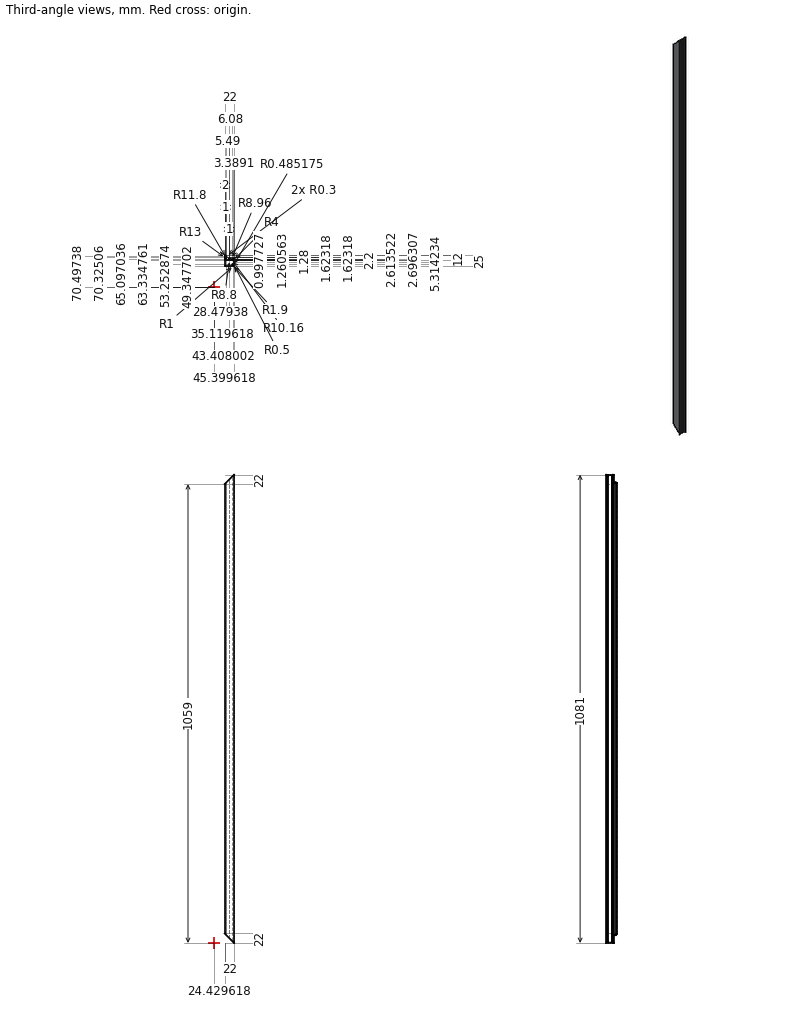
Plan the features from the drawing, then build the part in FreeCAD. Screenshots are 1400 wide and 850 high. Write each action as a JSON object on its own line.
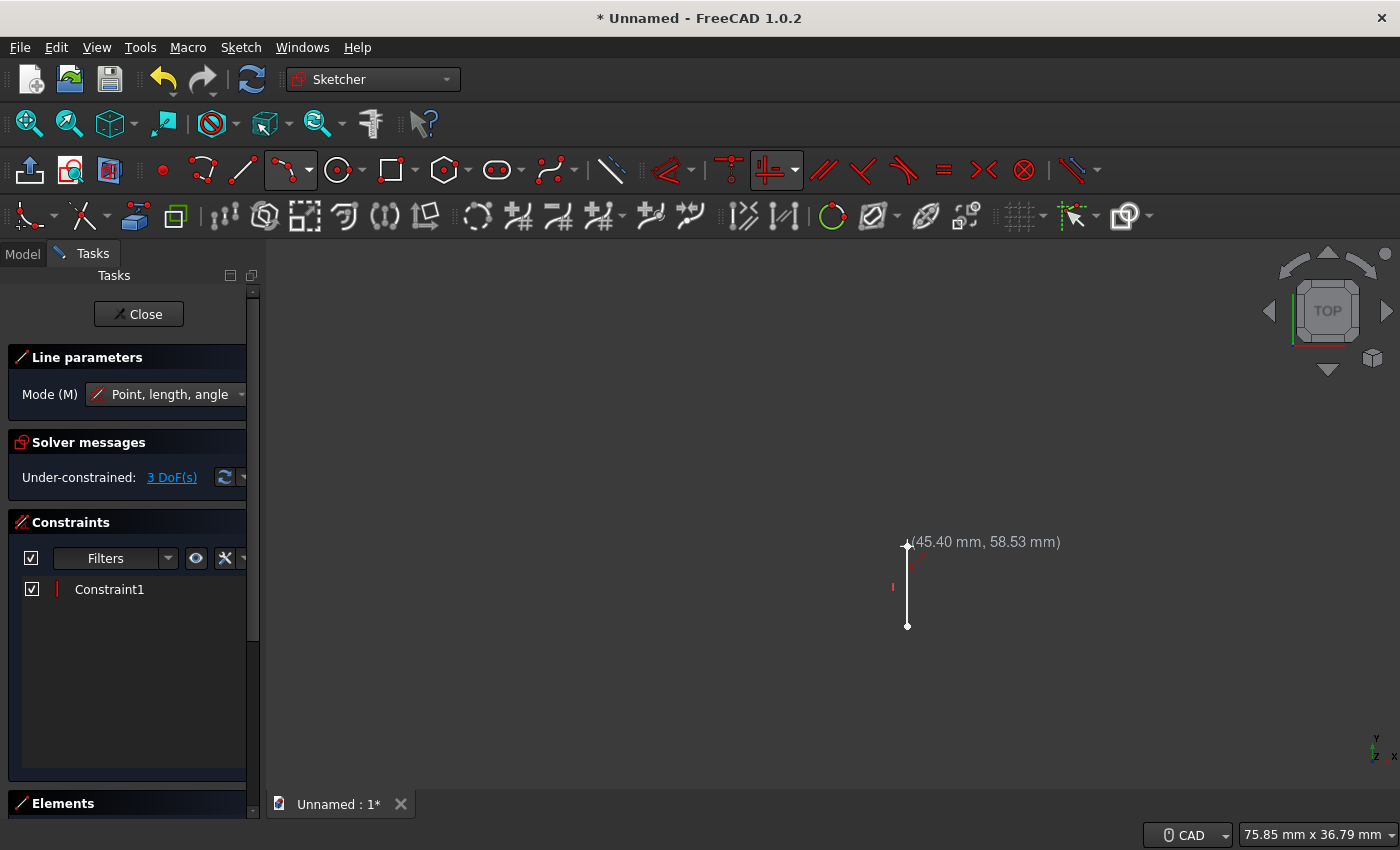
{"action": "left_click", "coordinate": [204, 170]}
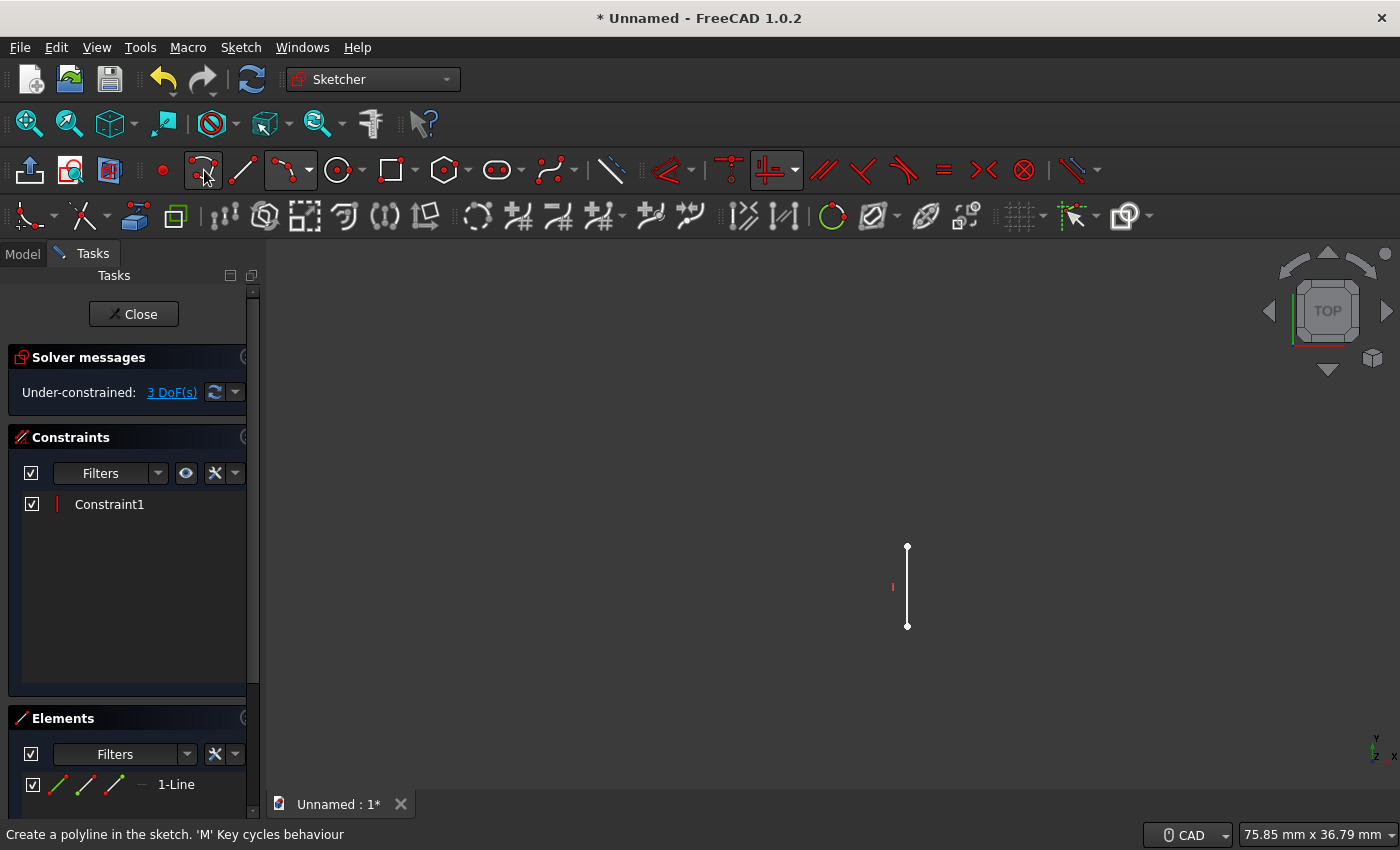
{"action": "left_click", "coordinate": [847, 487]}
{"action": "left_click", "coordinate": [756, 487]}
{"action": "left_click", "coordinate": [756, 472]}
{"action": "right_click", "coordinate": [756, 472]}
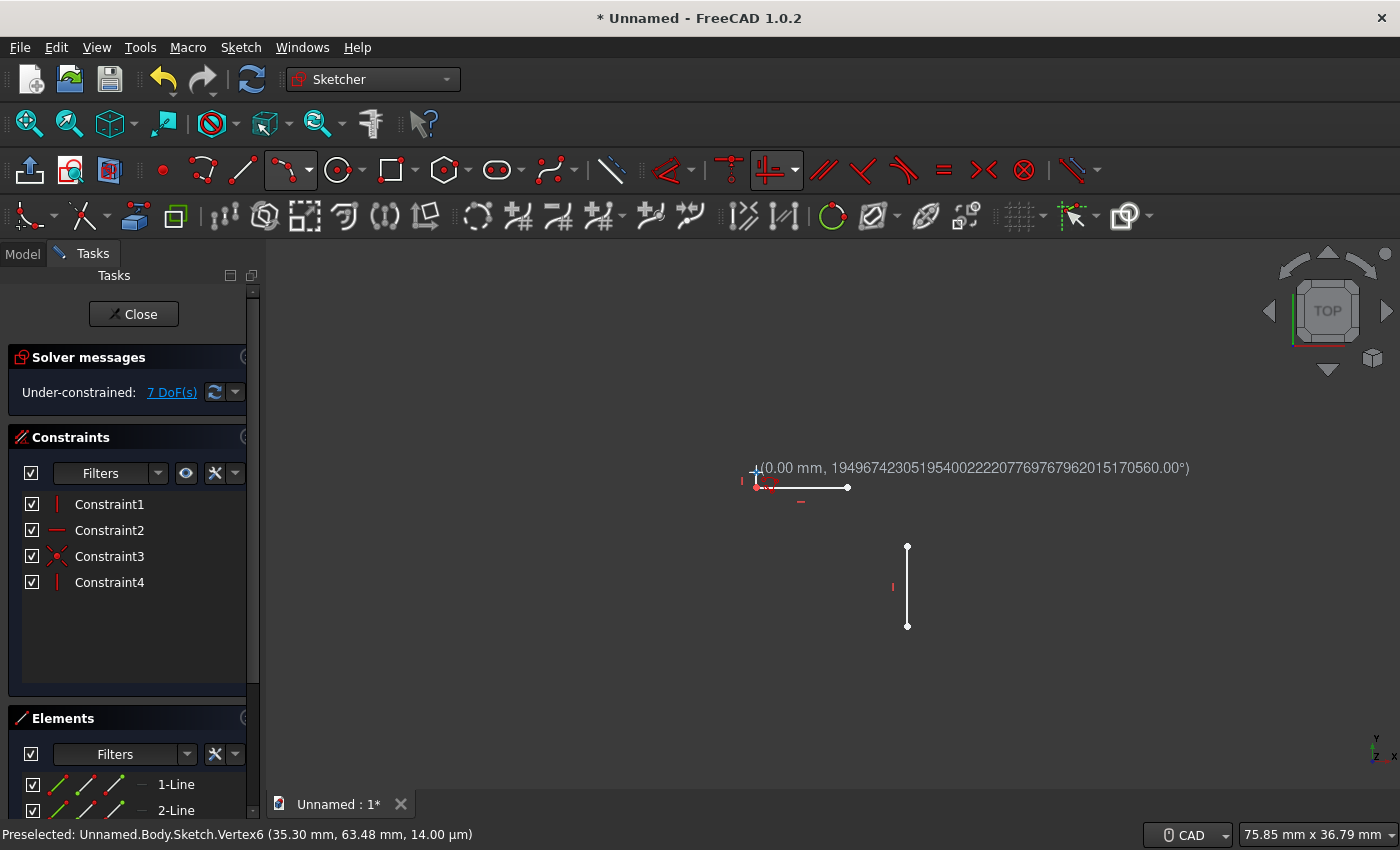
{"action": "left_click", "coordinate": [877, 475]}
{"action": "left_click", "coordinate": [922, 461]}
{"action": "left_click", "coordinate": [922, 442]}
{"action": "left_click", "coordinate": [872, 458]}
{"action": "right_click", "coordinate": [872, 458]}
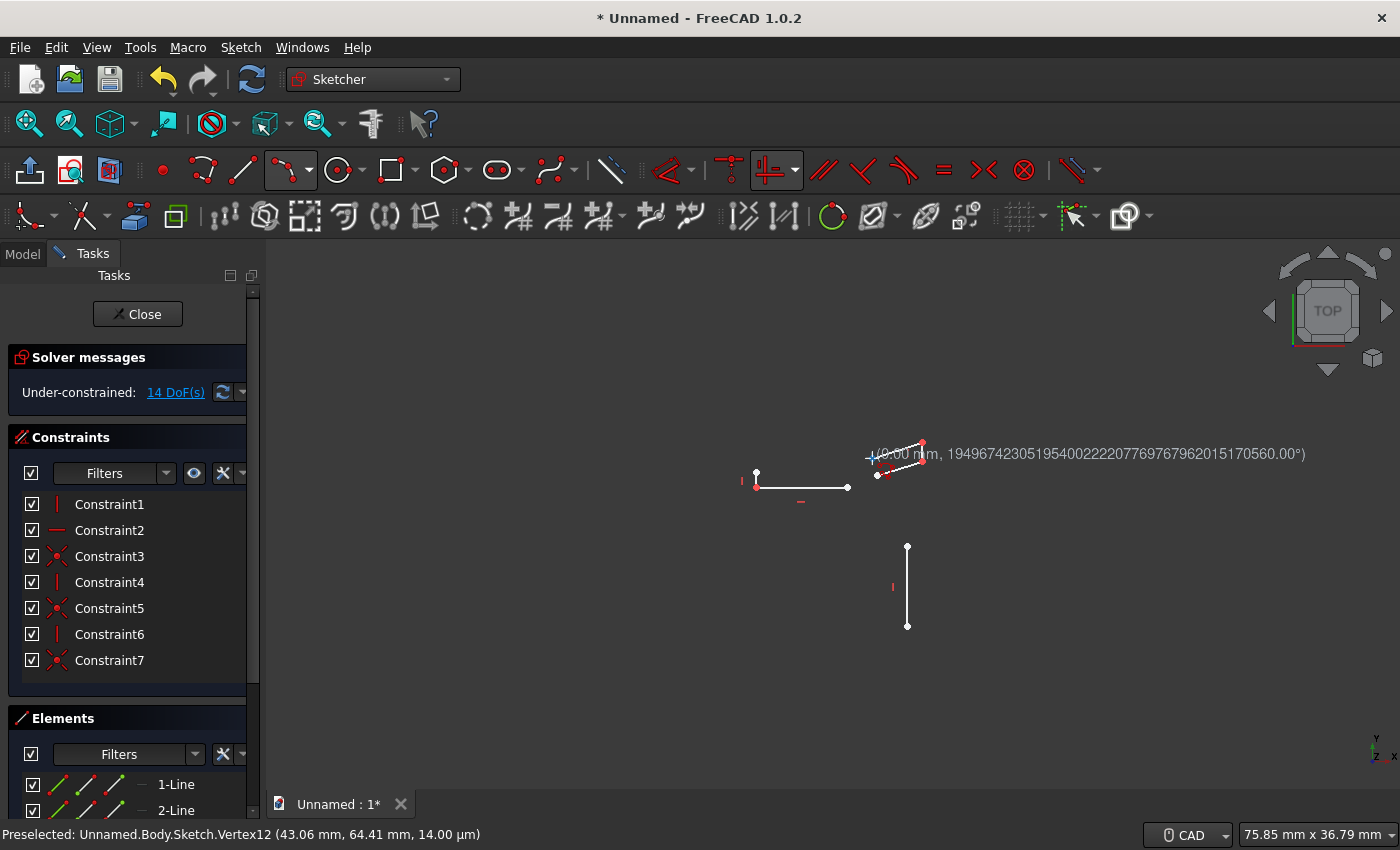
{"action": "left_click", "coordinate": [753, 454]}
{"action": "left_click", "coordinate": [738, 454]}
{"action": "left_click", "coordinate": [738, 487]}
{"action": "left_click", "coordinate": [656, 487]}
{"action": "left_click", "coordinate": [651, 446]}
{"action": "right_click", "coordinate": [651, 446]}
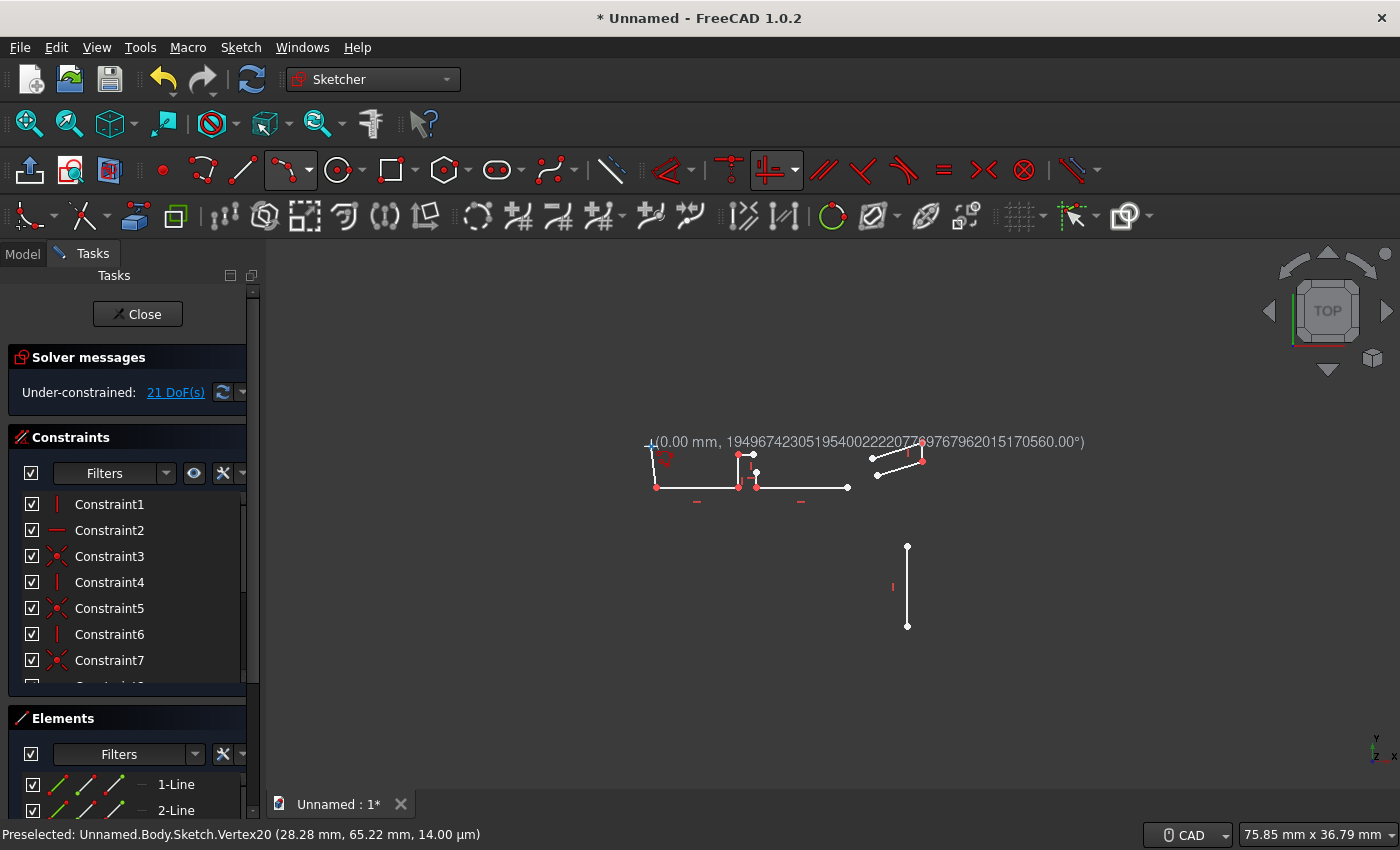
{"action": "left_click", "coordinate": [244, 170]}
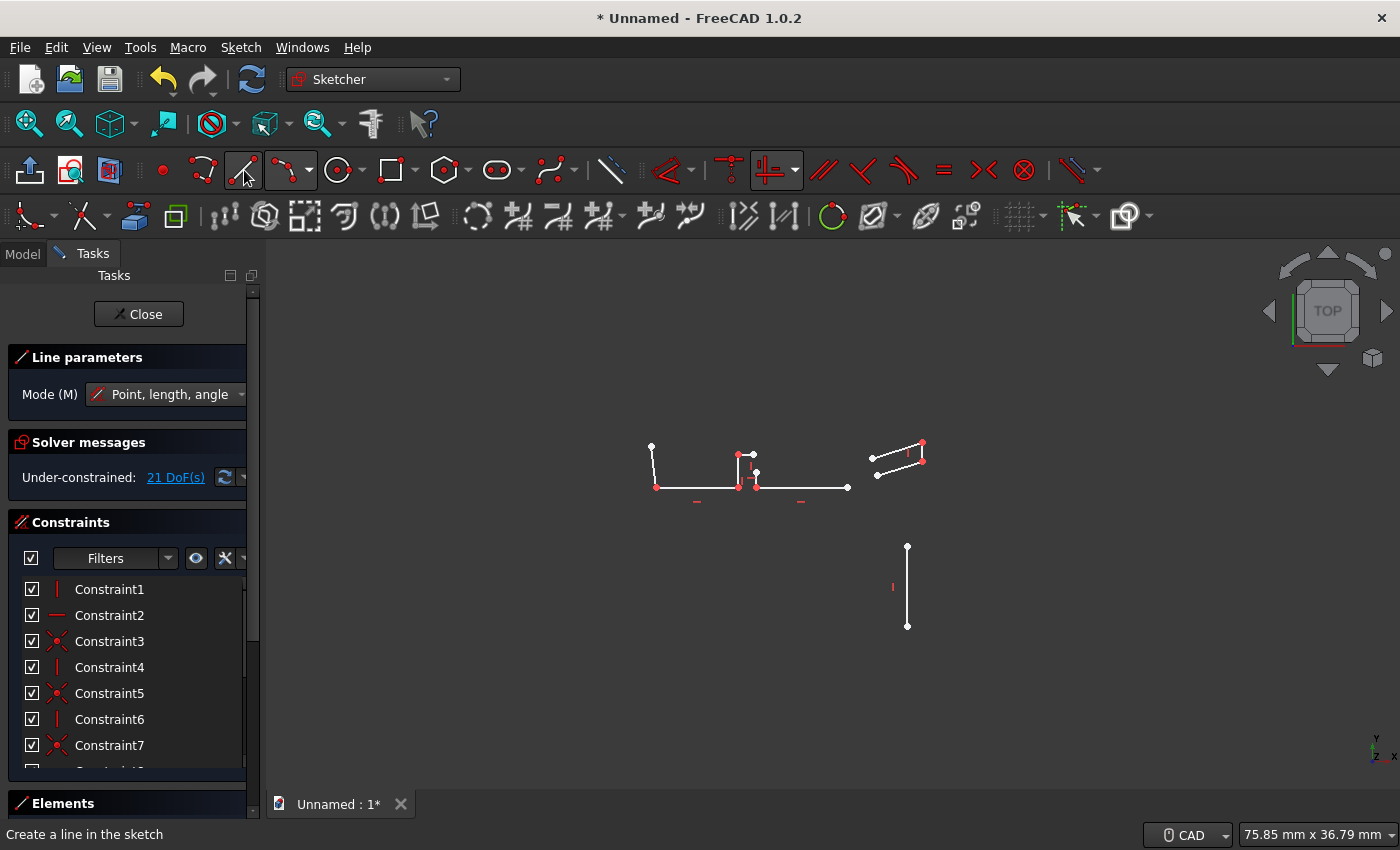
{"action": "left_click", "coordinate": [651, 397]}
{"action": "left_click", "coordinate": [654, 373]}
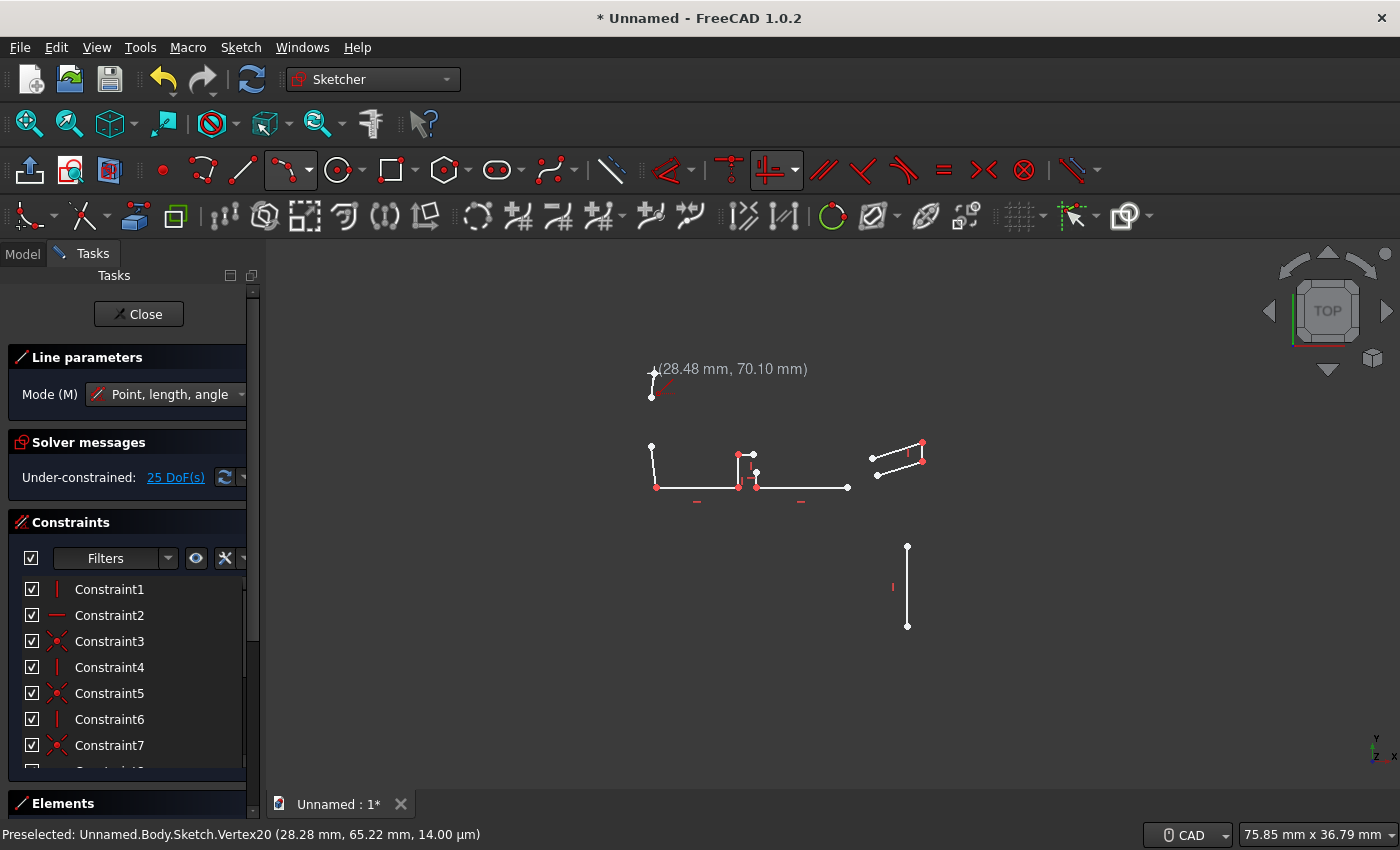
{"action": "scroll", "coordinate": [650, 368], "scroll_direction": "up", "scroll_amount": 5}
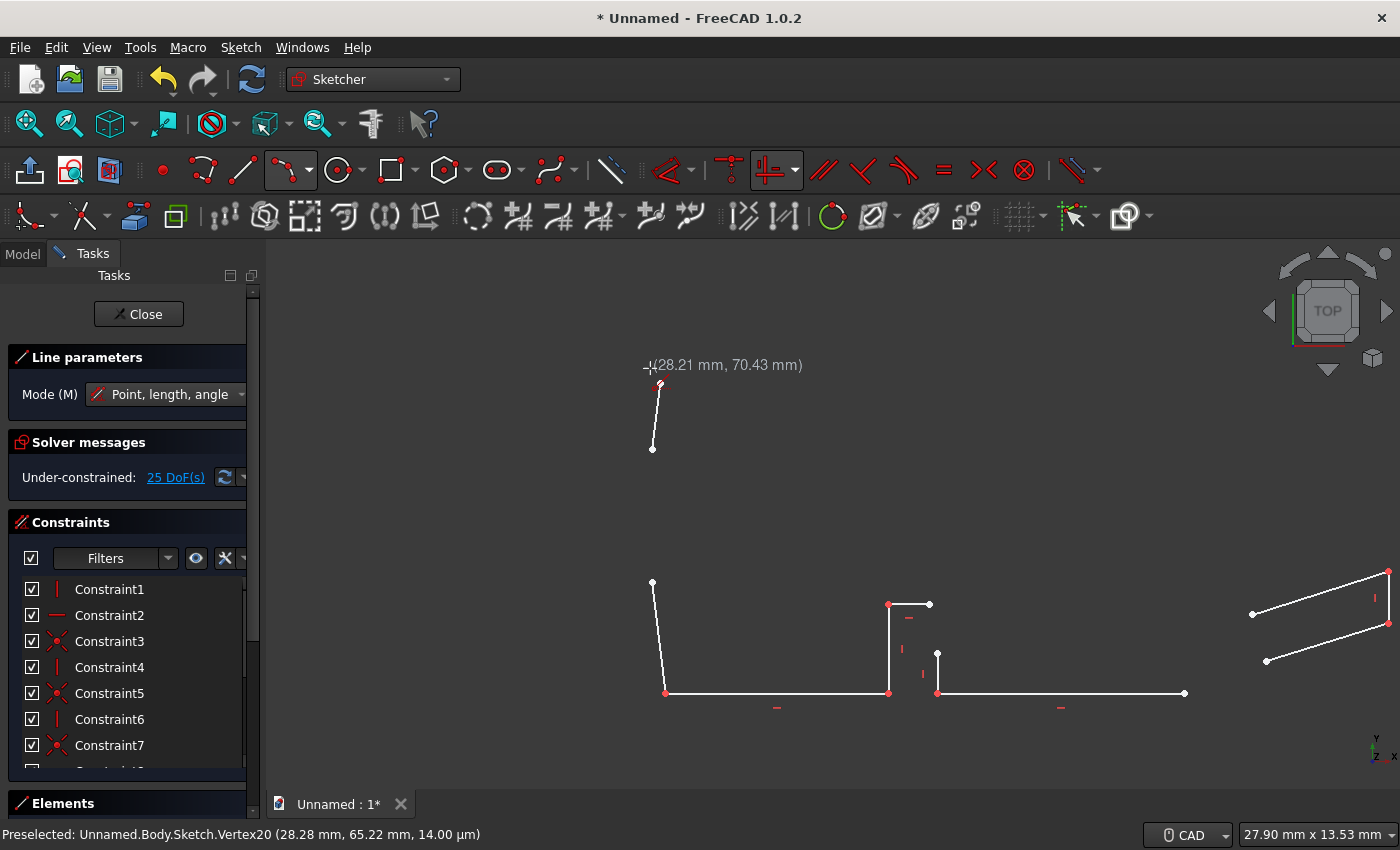
{"action": "left_click", "coordinate": [650, 368]}
{"action": "left_click", "coordinate": [626, 364]}